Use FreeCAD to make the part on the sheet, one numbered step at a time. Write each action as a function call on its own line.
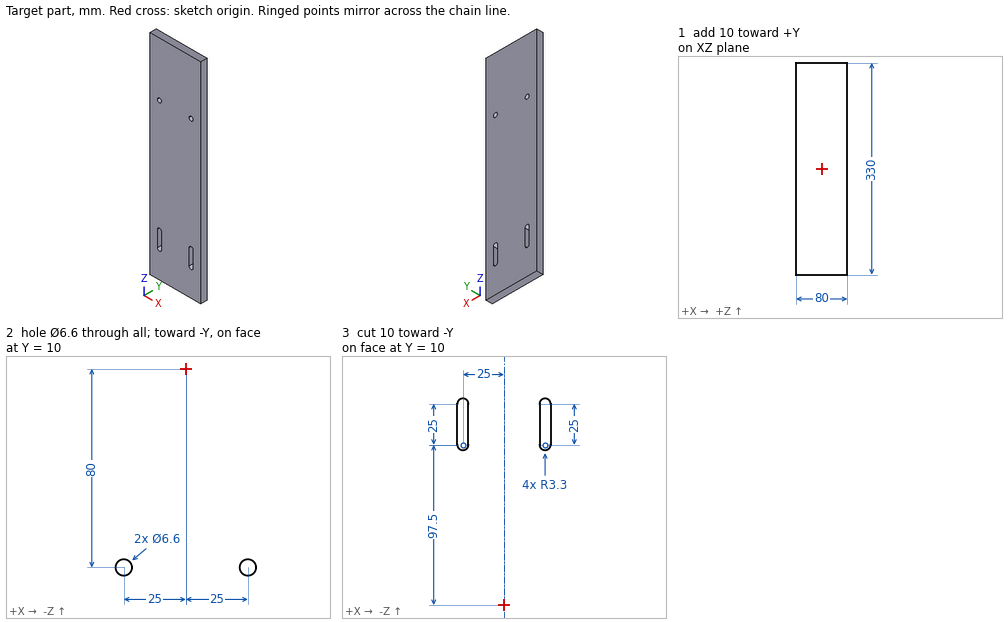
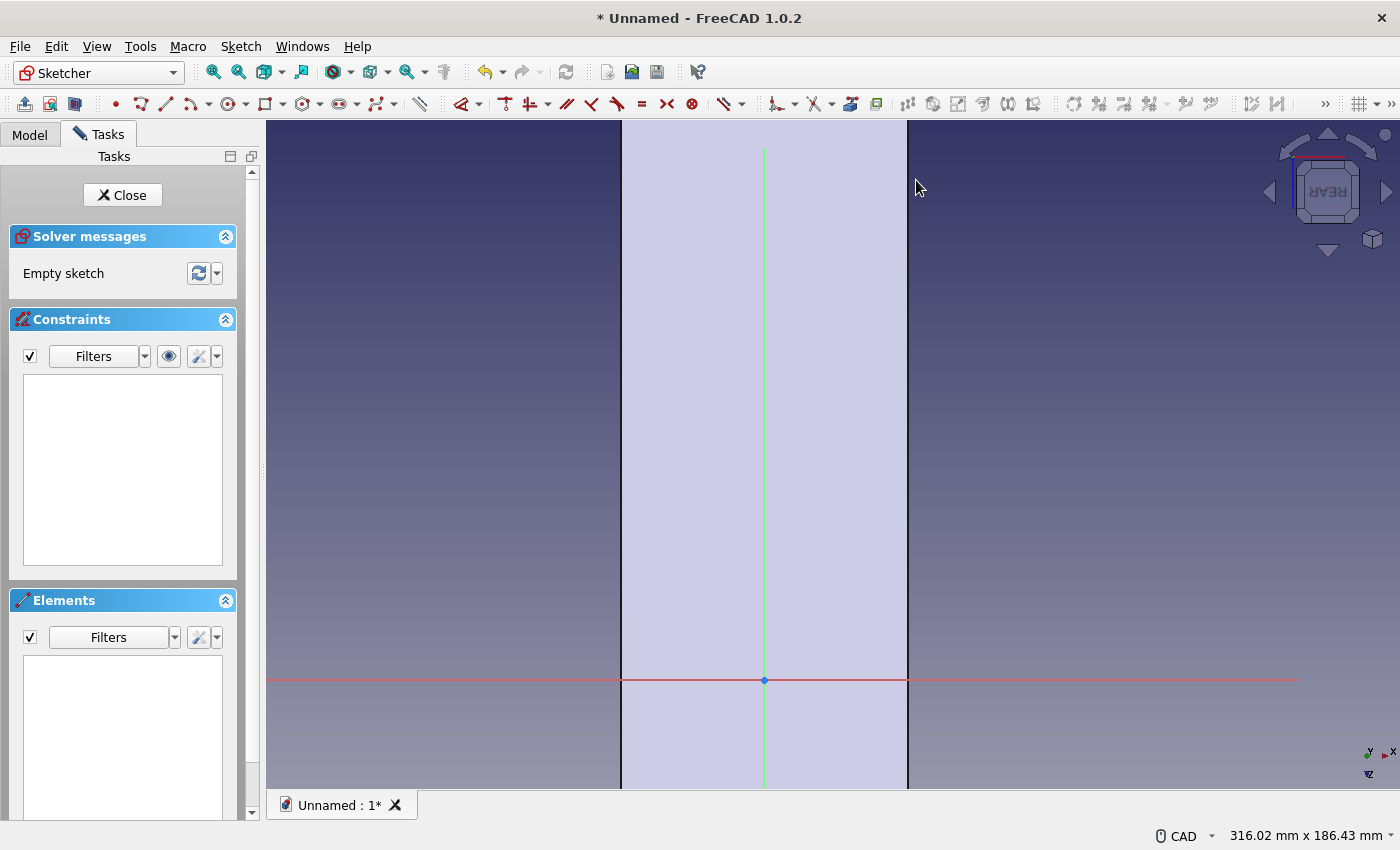
scroll(675, 330, up, 4)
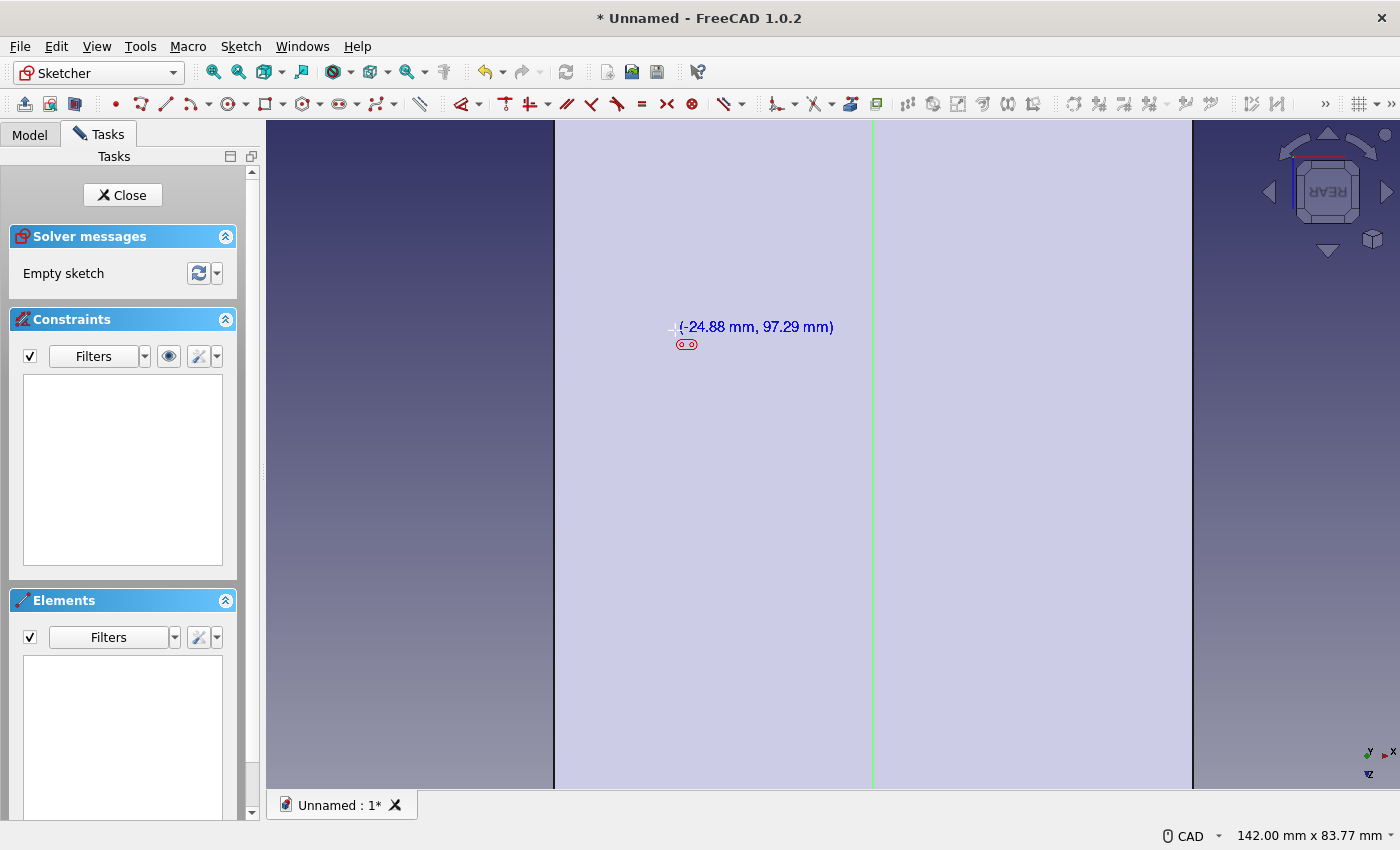
click(674, 330)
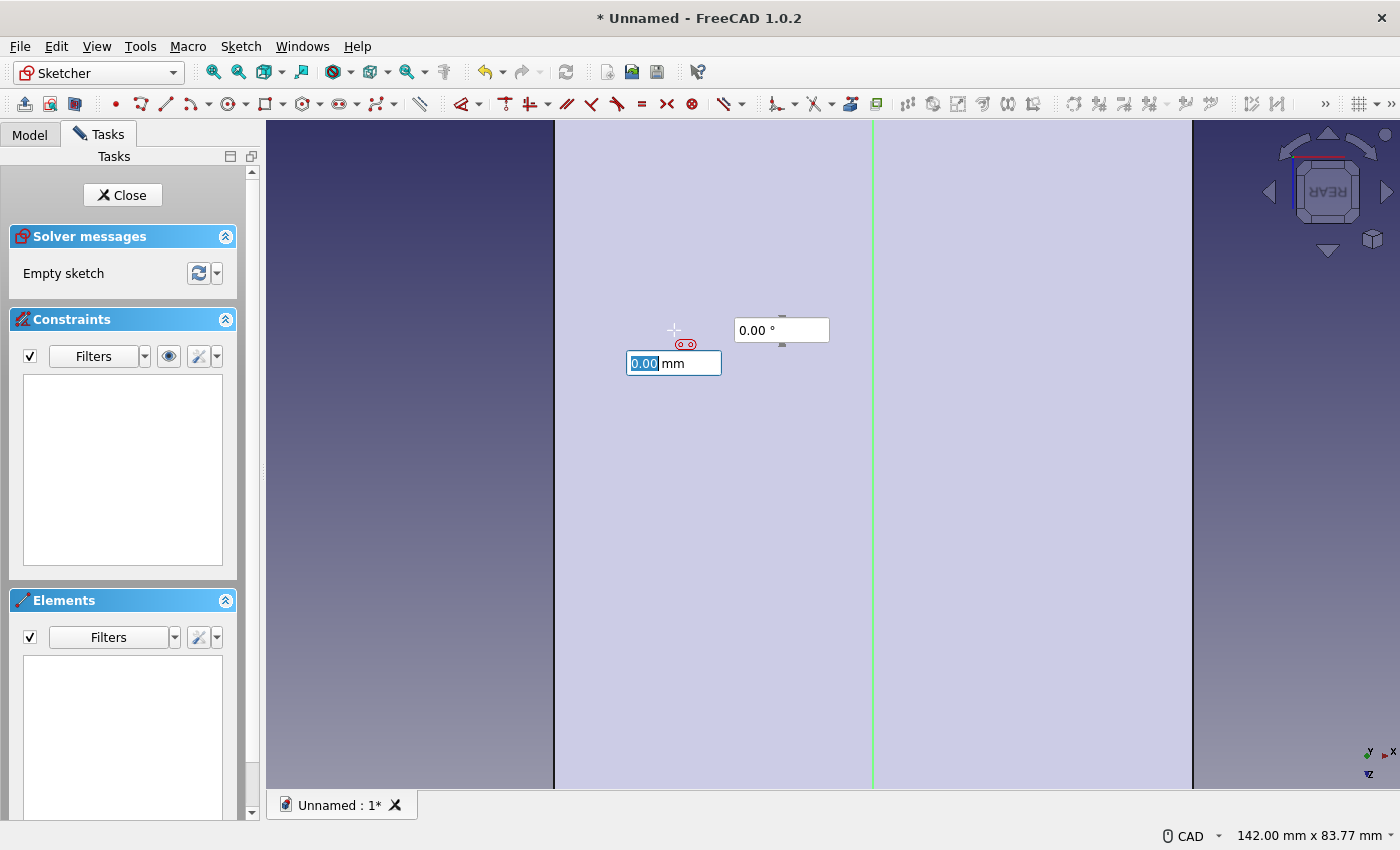
scroll(676, 331, down, 4)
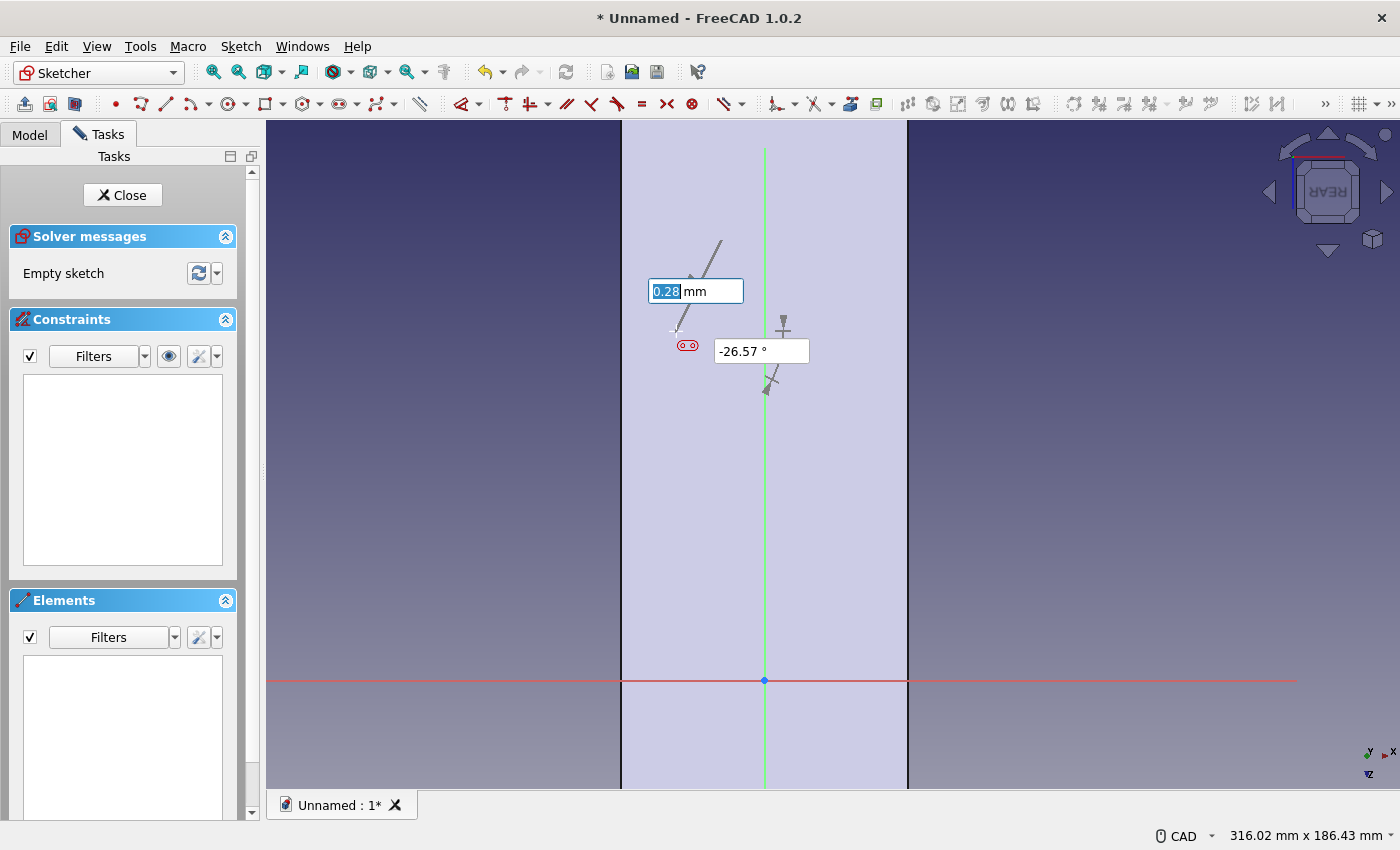
click(675, 241)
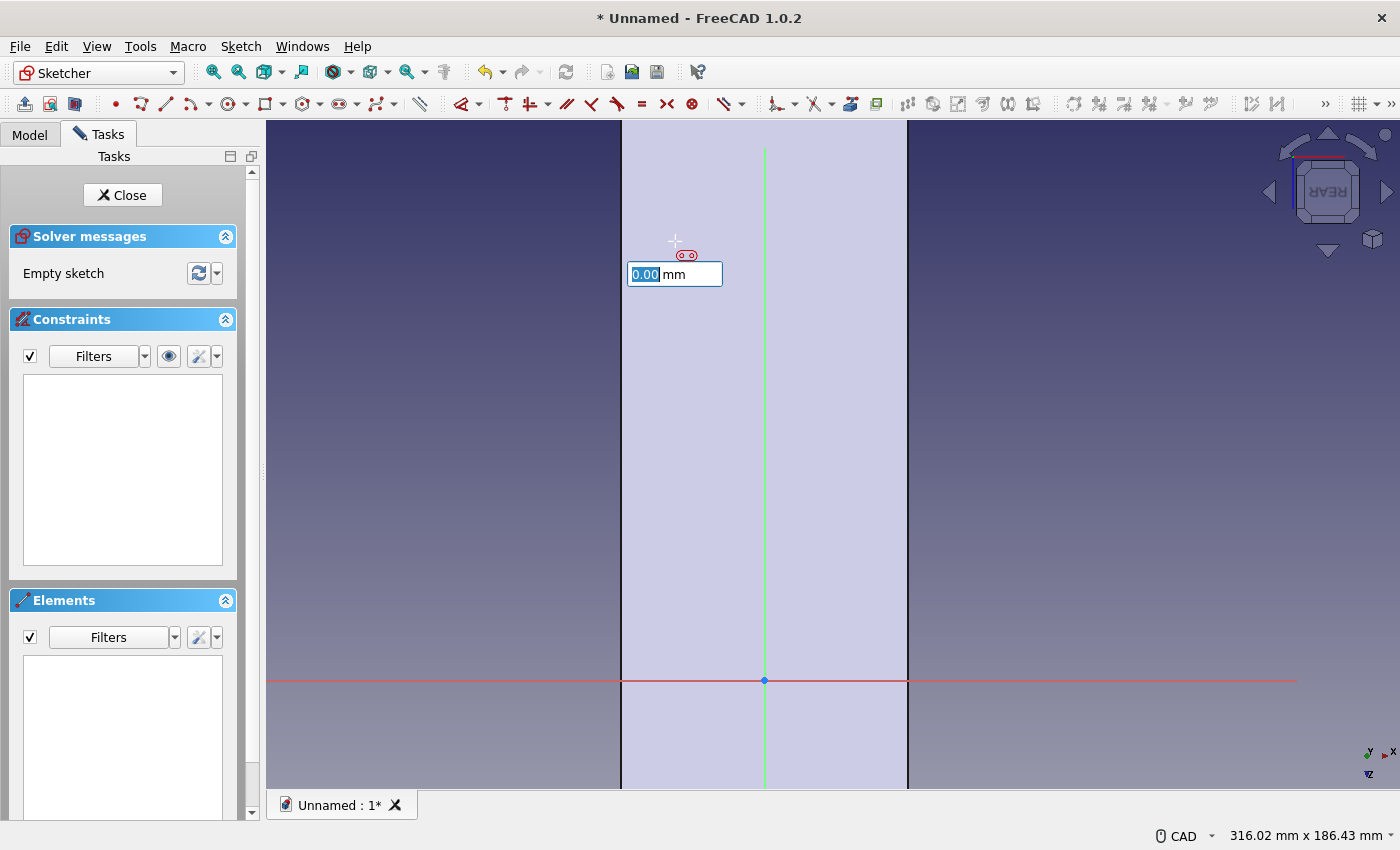
scroll(663, 286, up, 2)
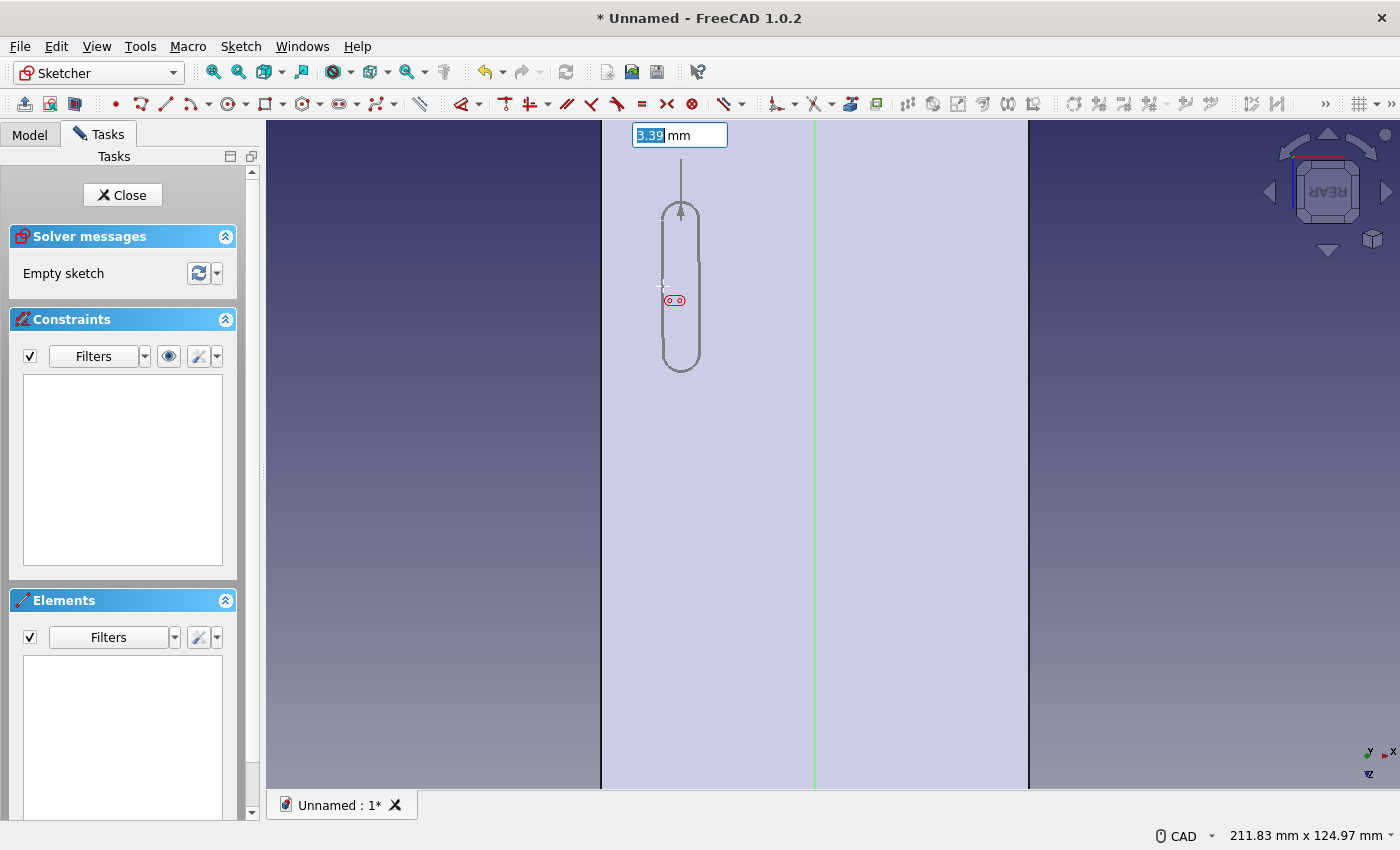
click(663, 286)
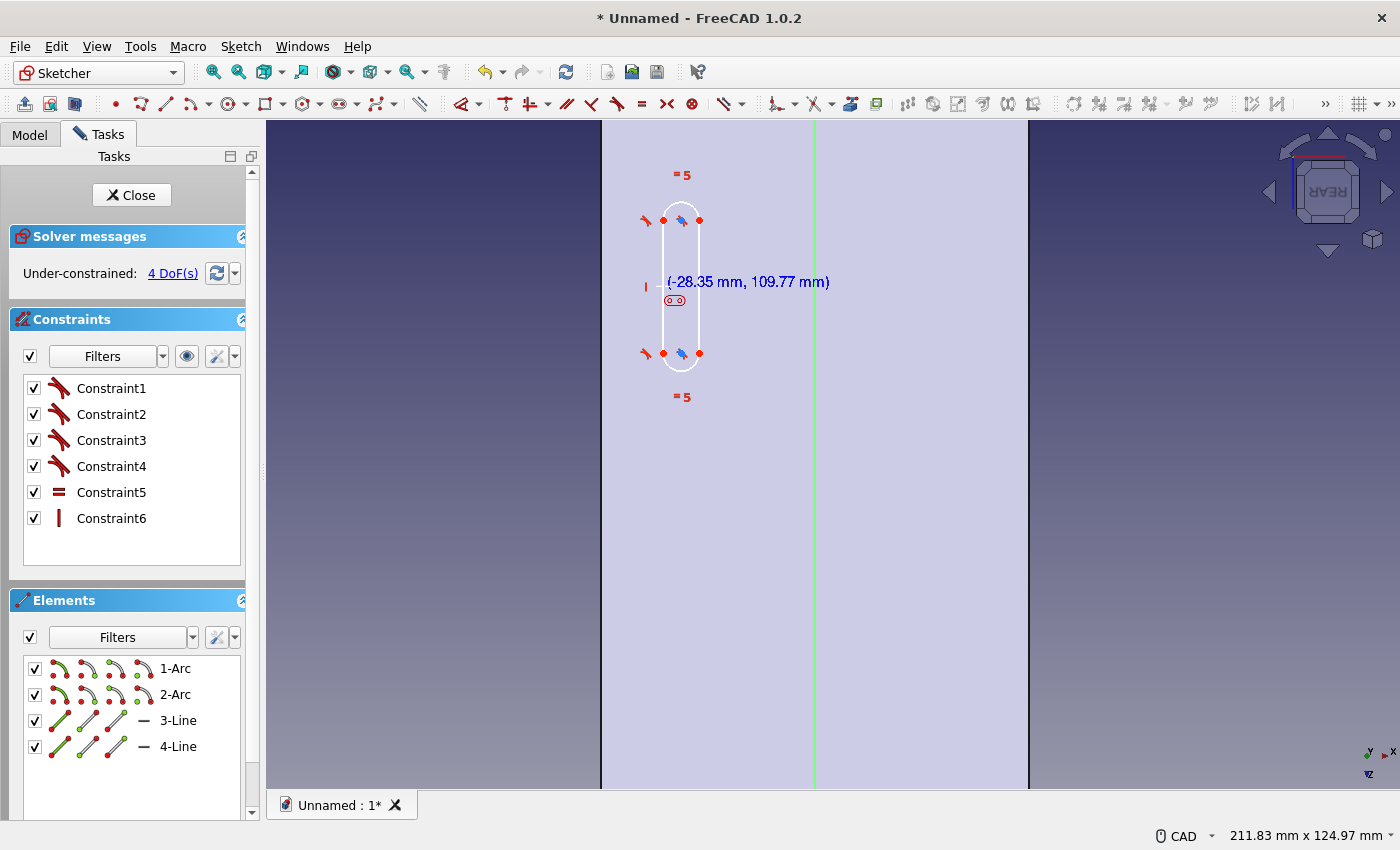
scroll(949, 353, up, 2)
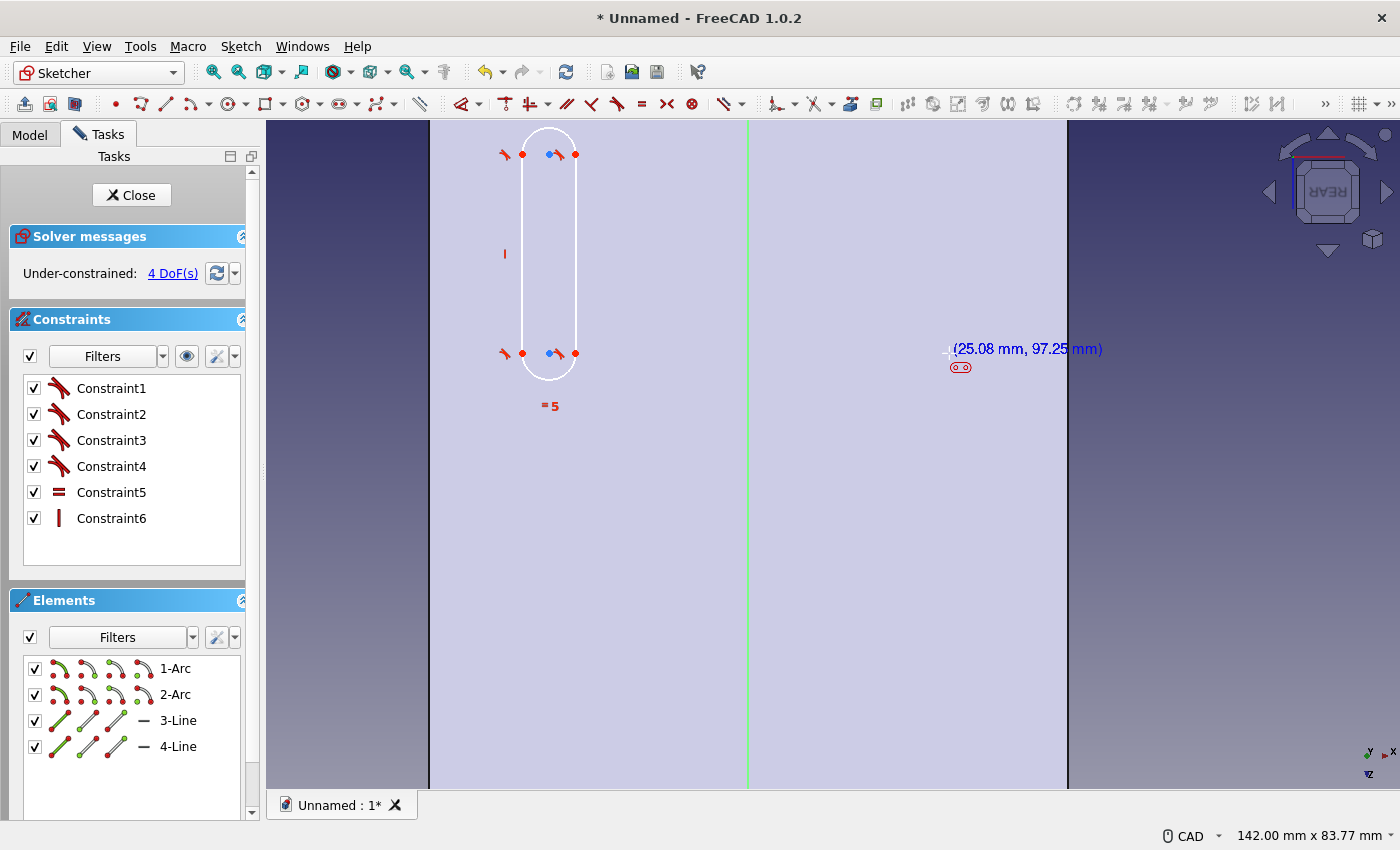
click(948, 352)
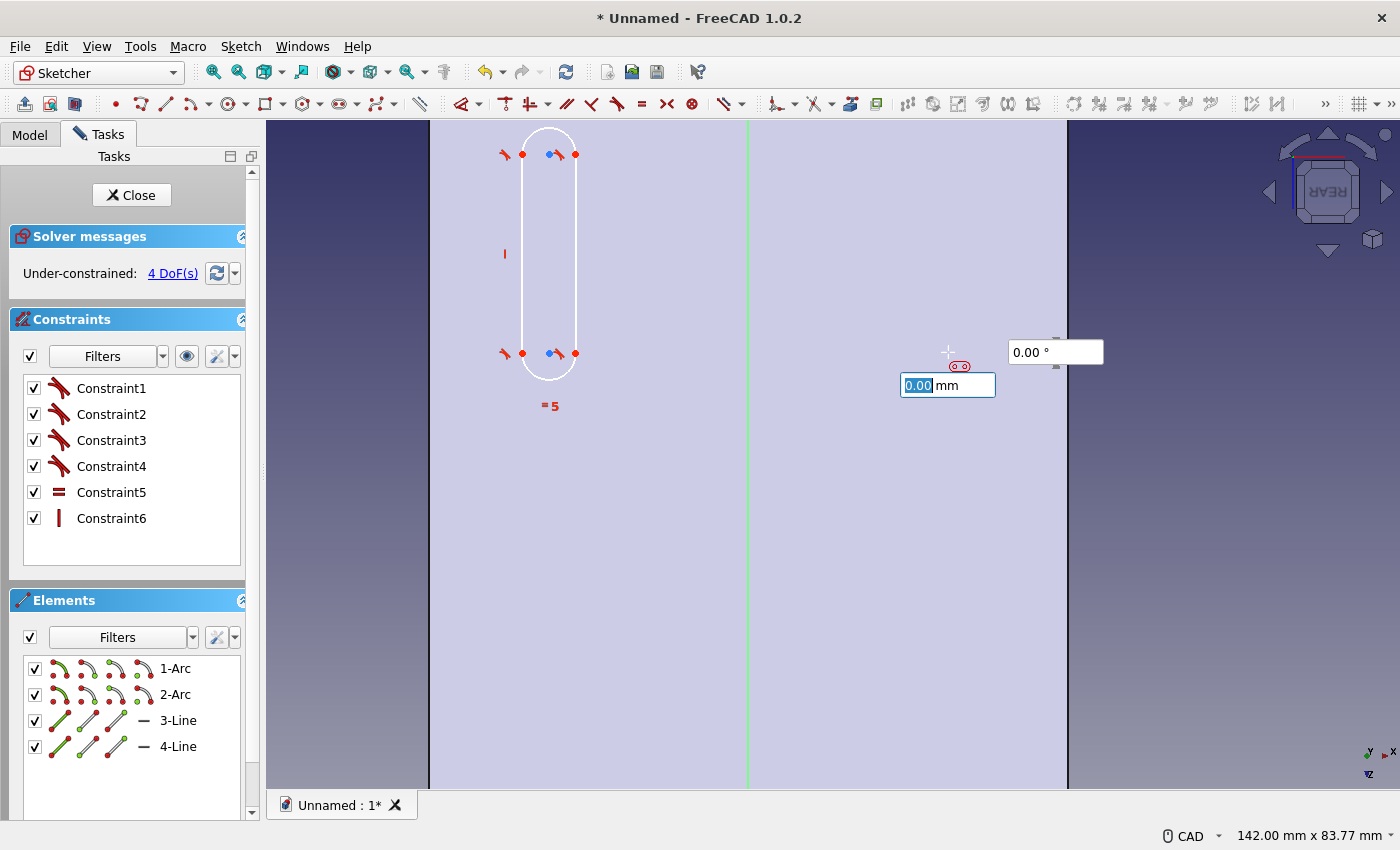
click(948, 153)